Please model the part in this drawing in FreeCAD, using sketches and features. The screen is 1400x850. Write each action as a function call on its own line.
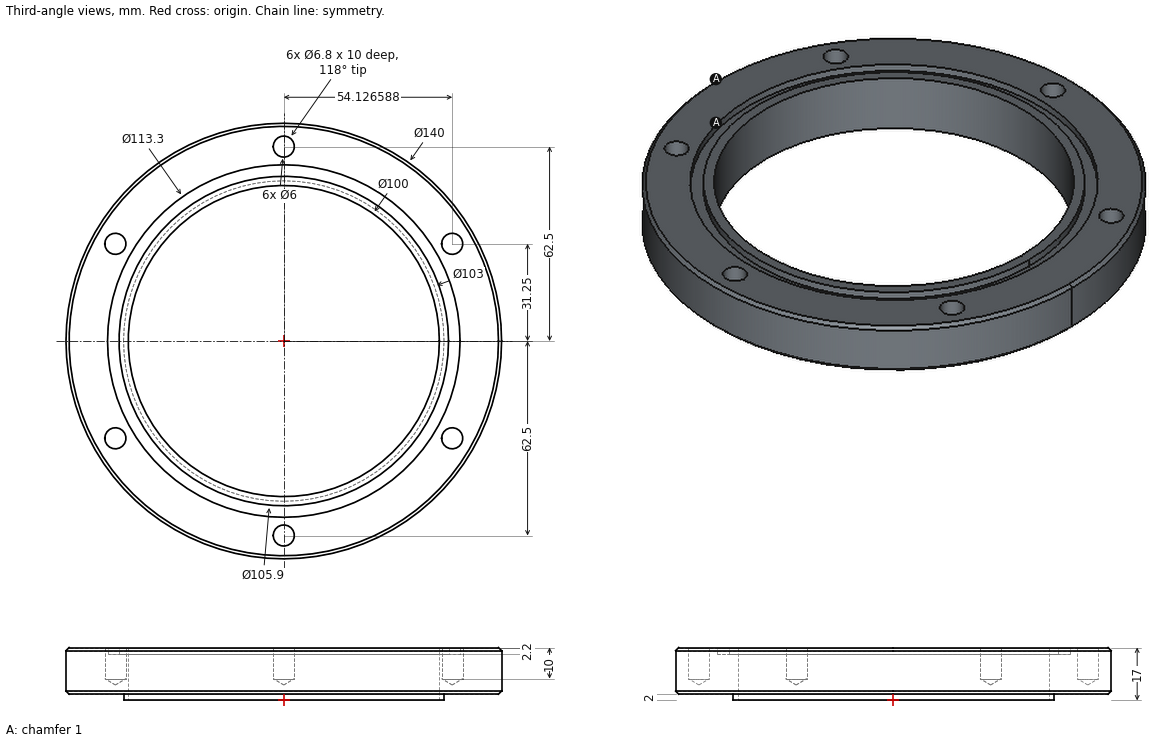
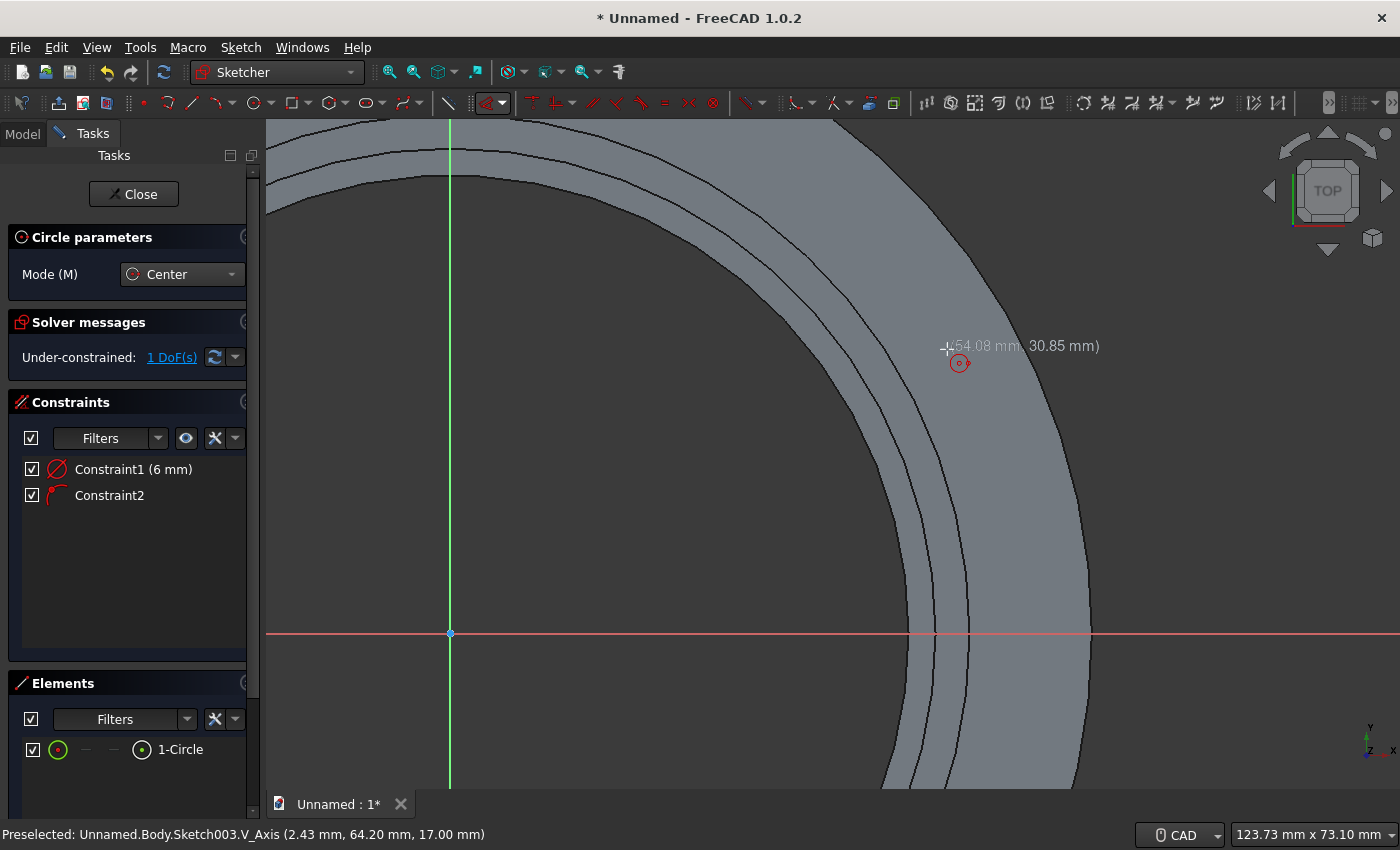
click(946, 347)
move(966, 328)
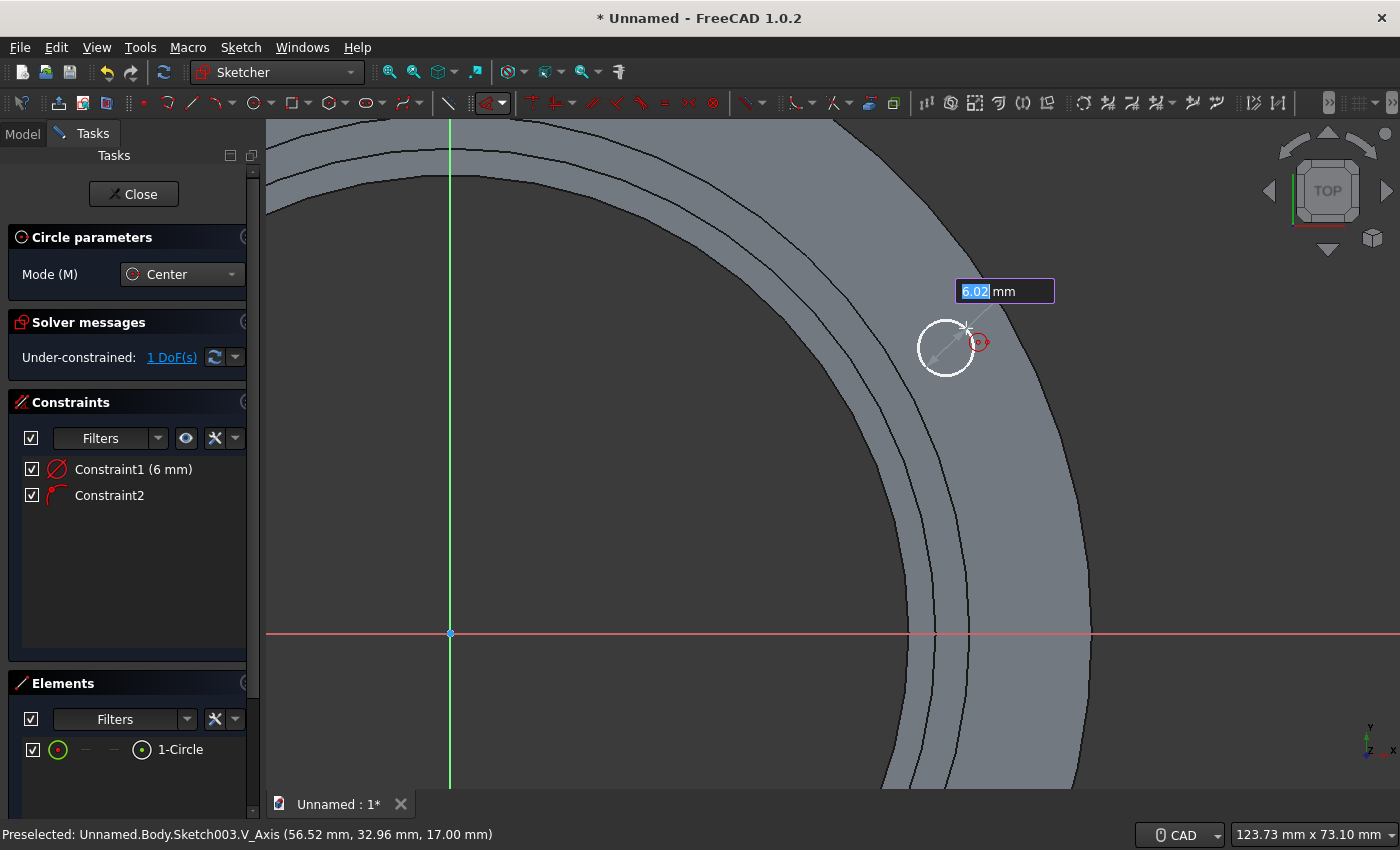
text(6)
key(Return)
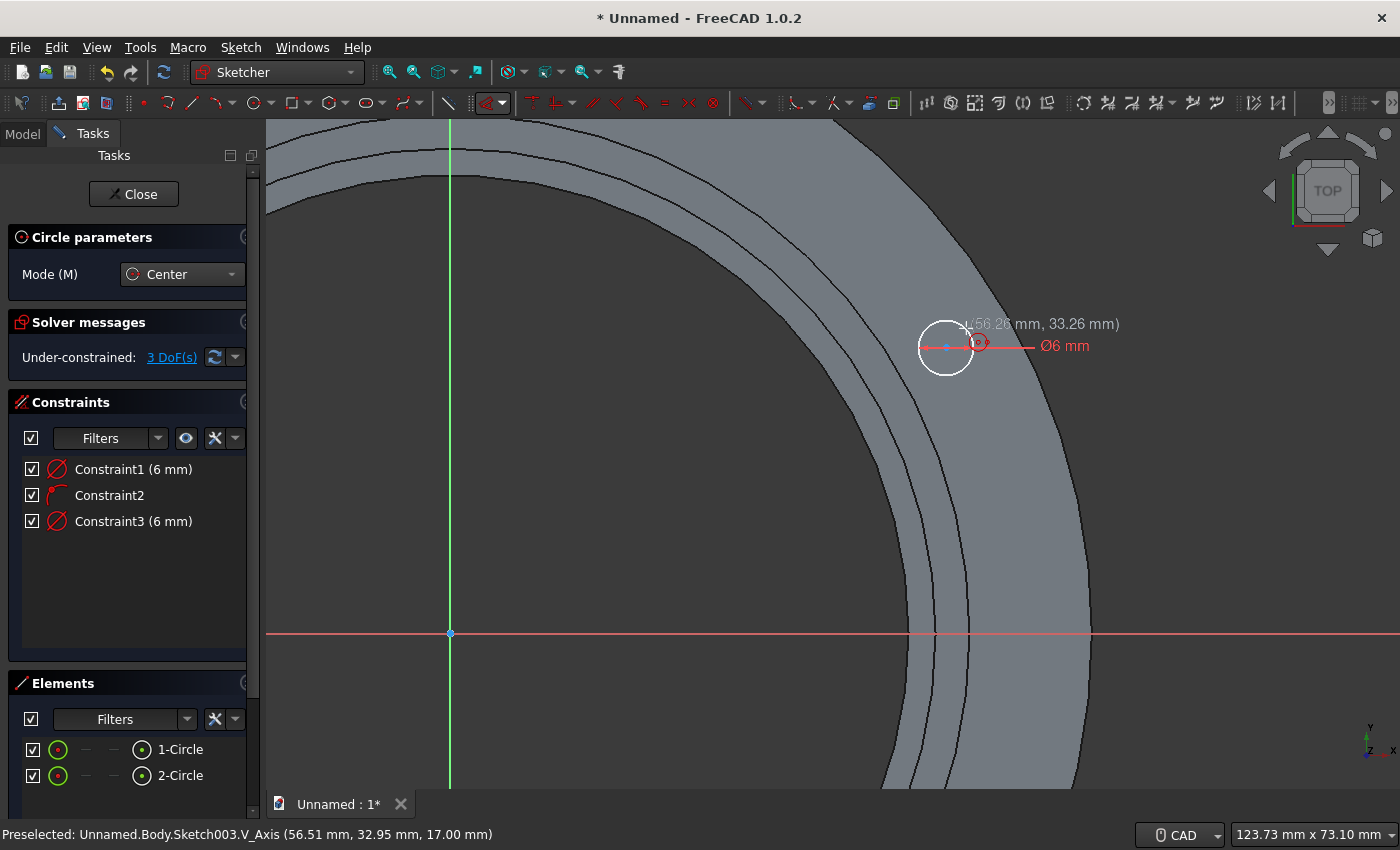
scroll(947, 349, down, 5)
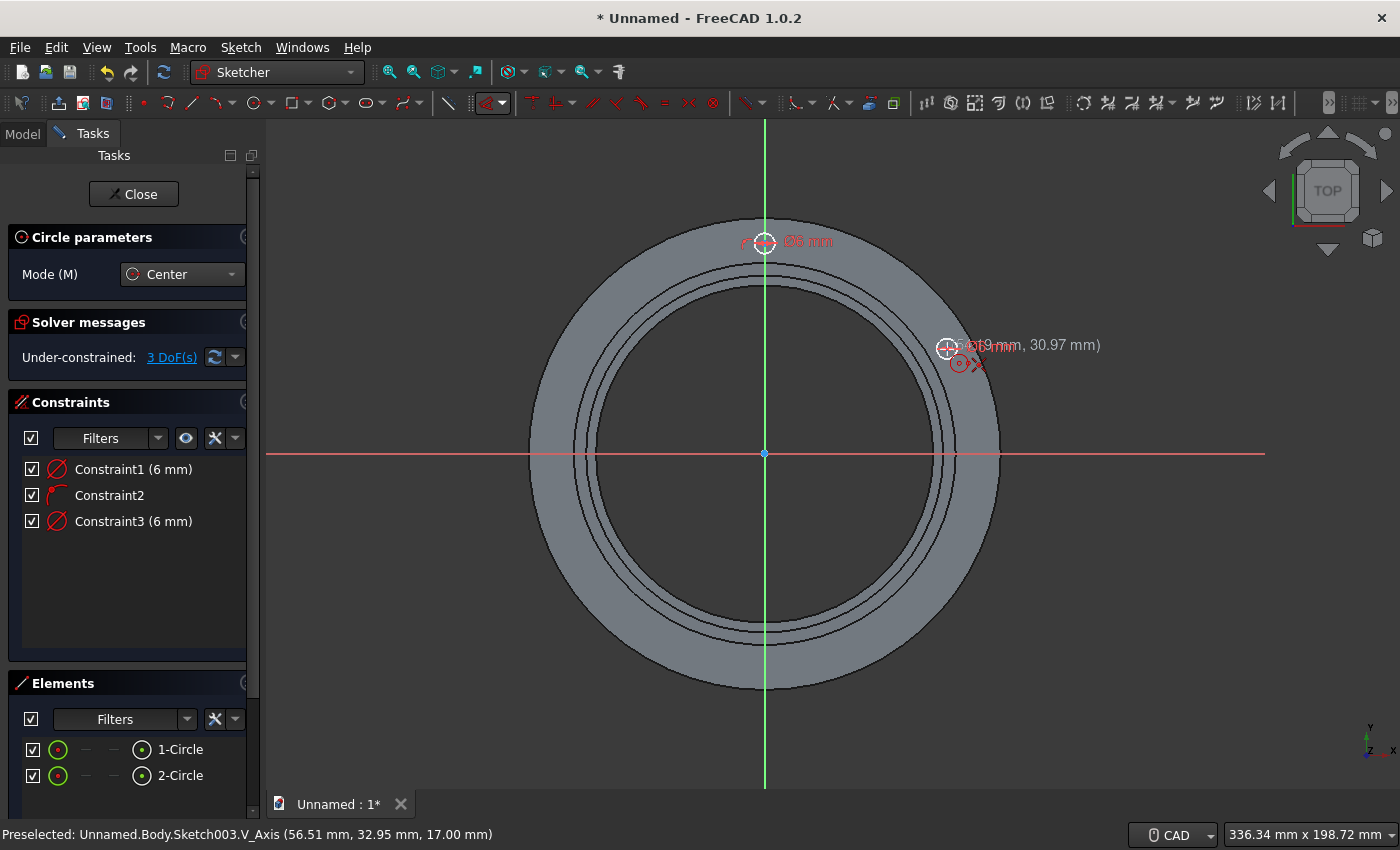
scroll(947, 559, up, 5)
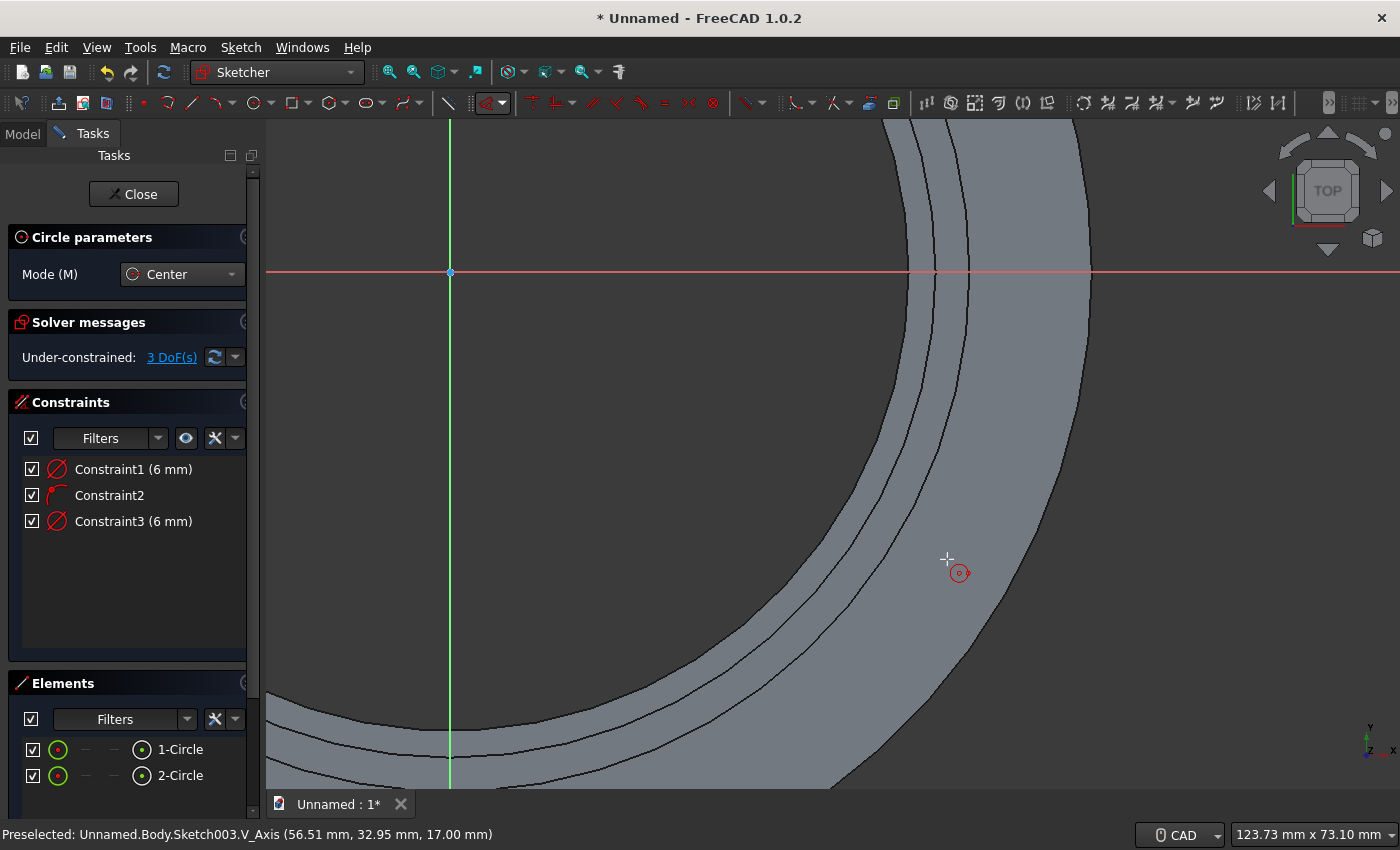
click(946, 559)
move(966, 539)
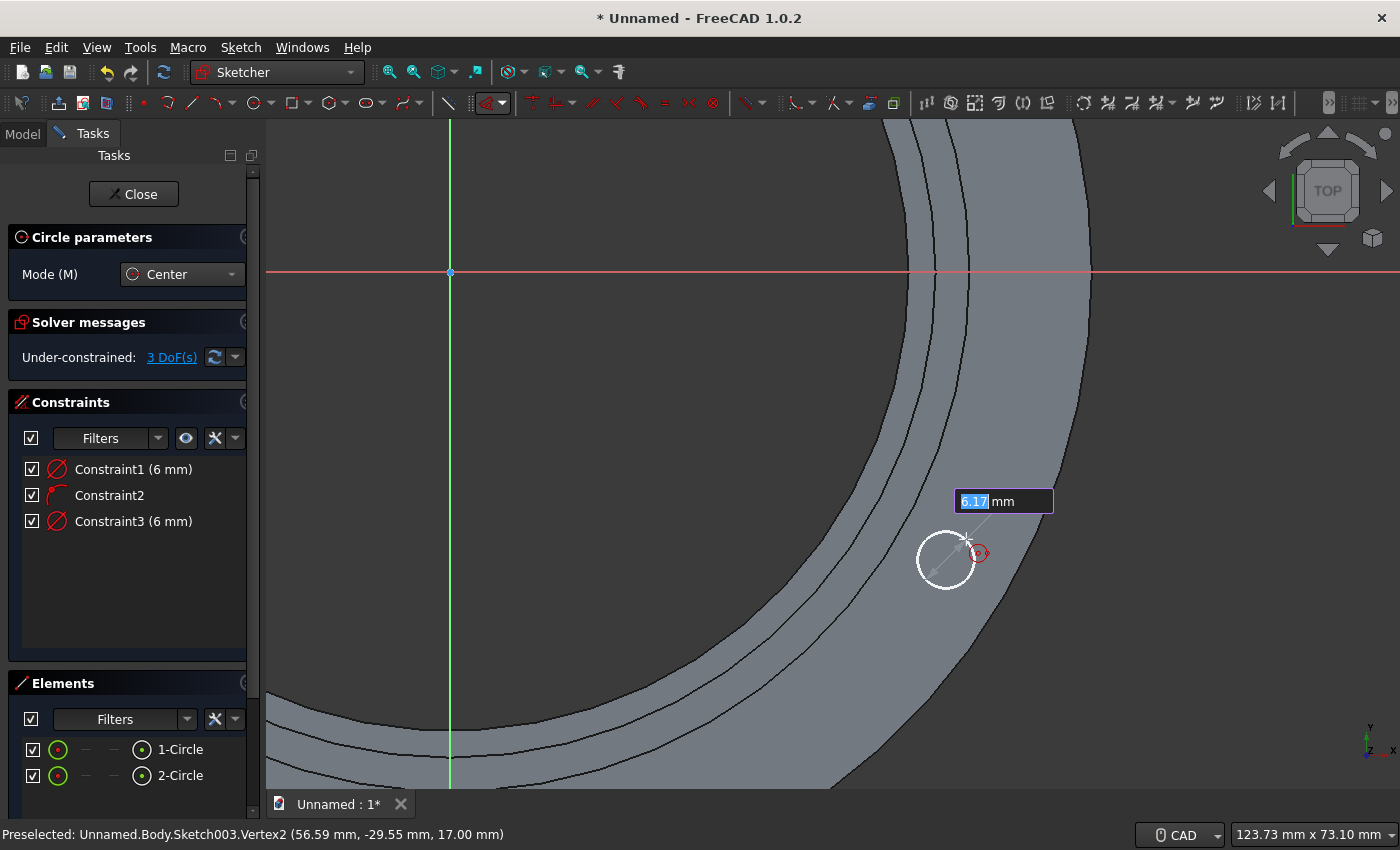
text(6)
key(Return)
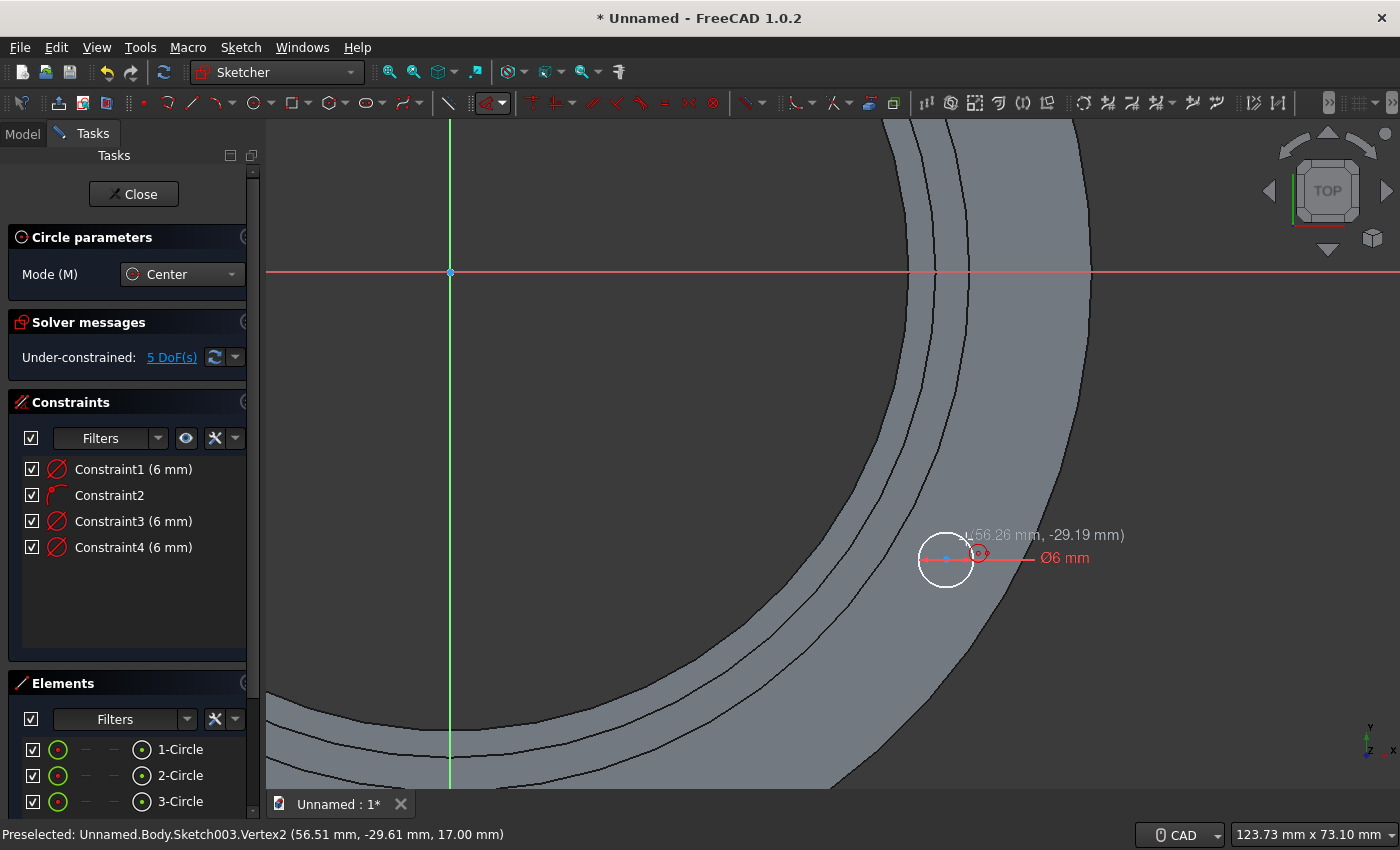
scroll(947, 560, down, 5)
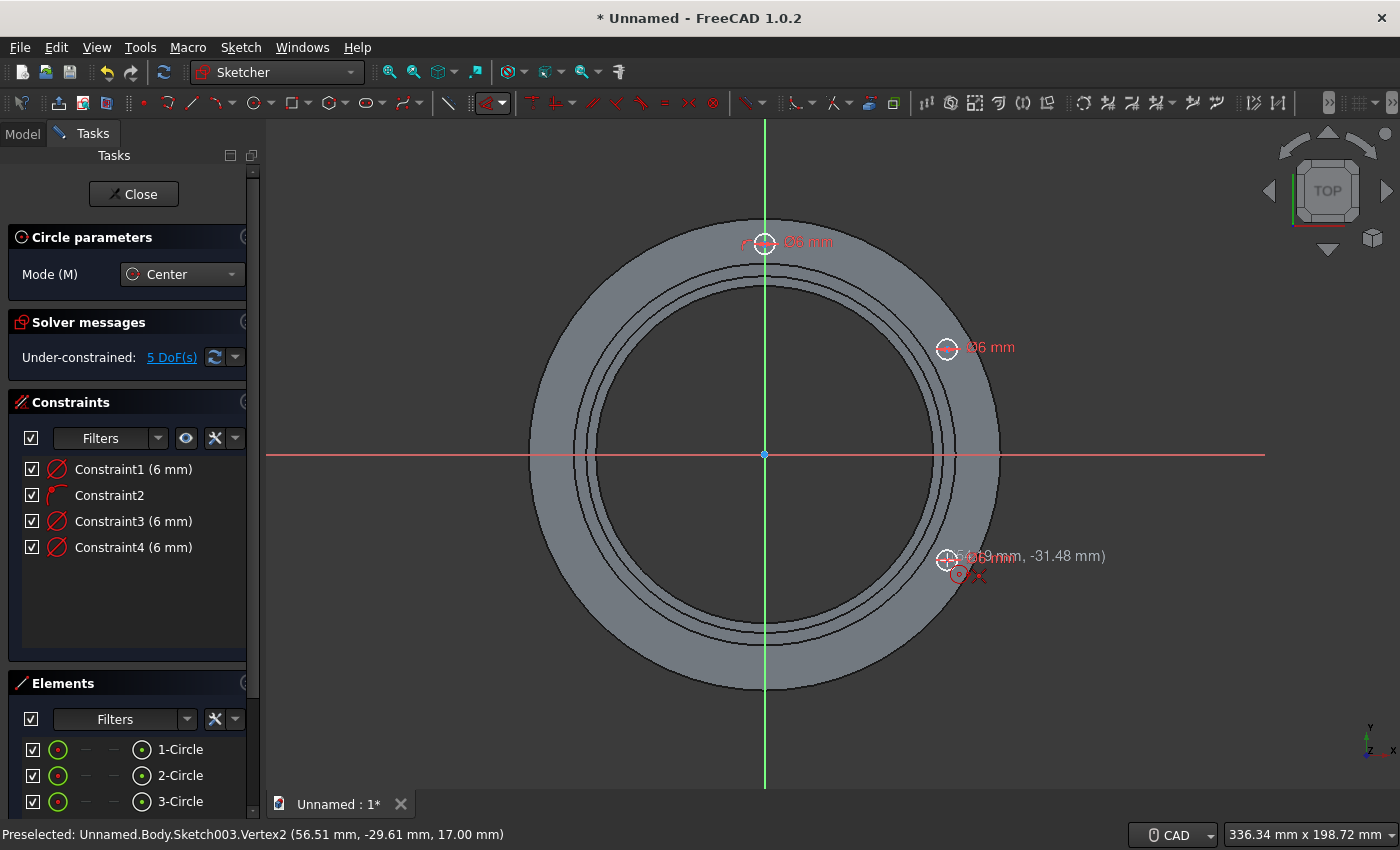
scroll(765, 665, up, 5)